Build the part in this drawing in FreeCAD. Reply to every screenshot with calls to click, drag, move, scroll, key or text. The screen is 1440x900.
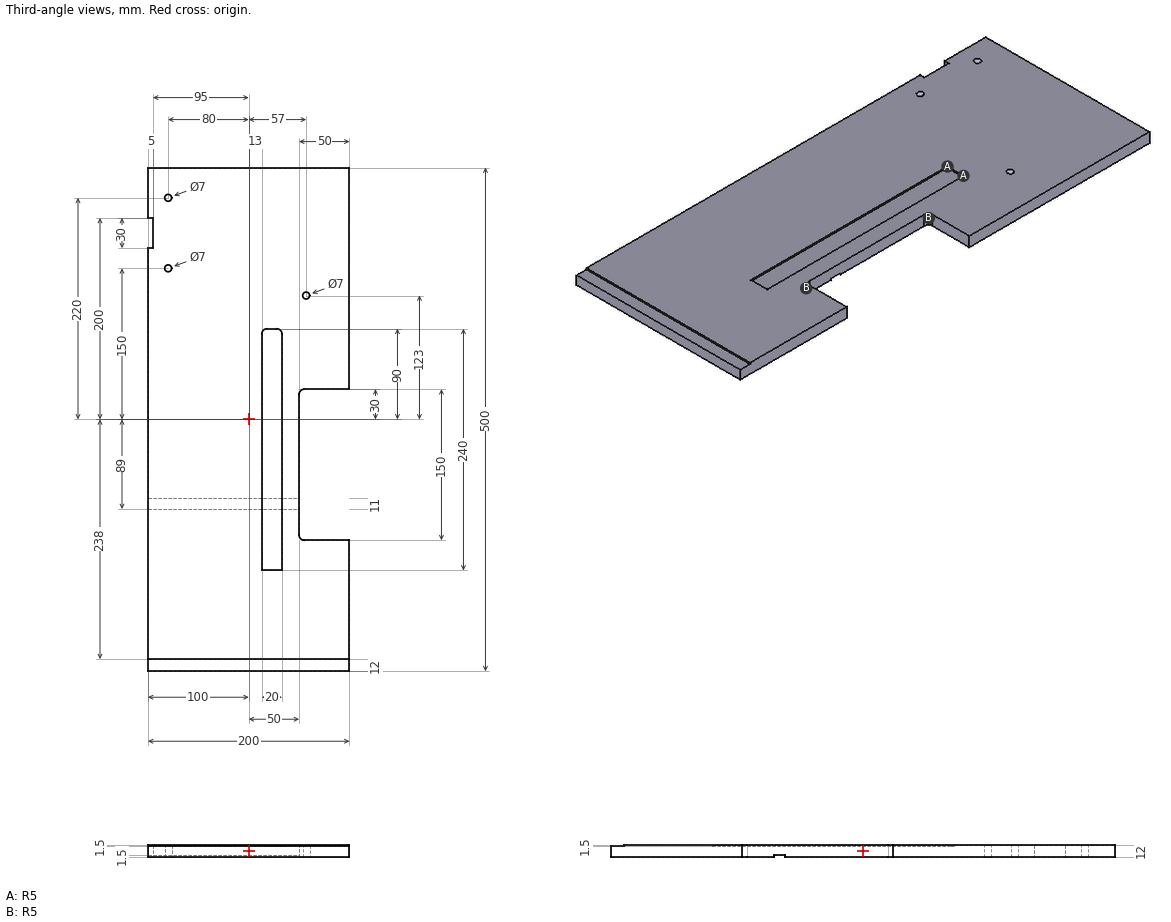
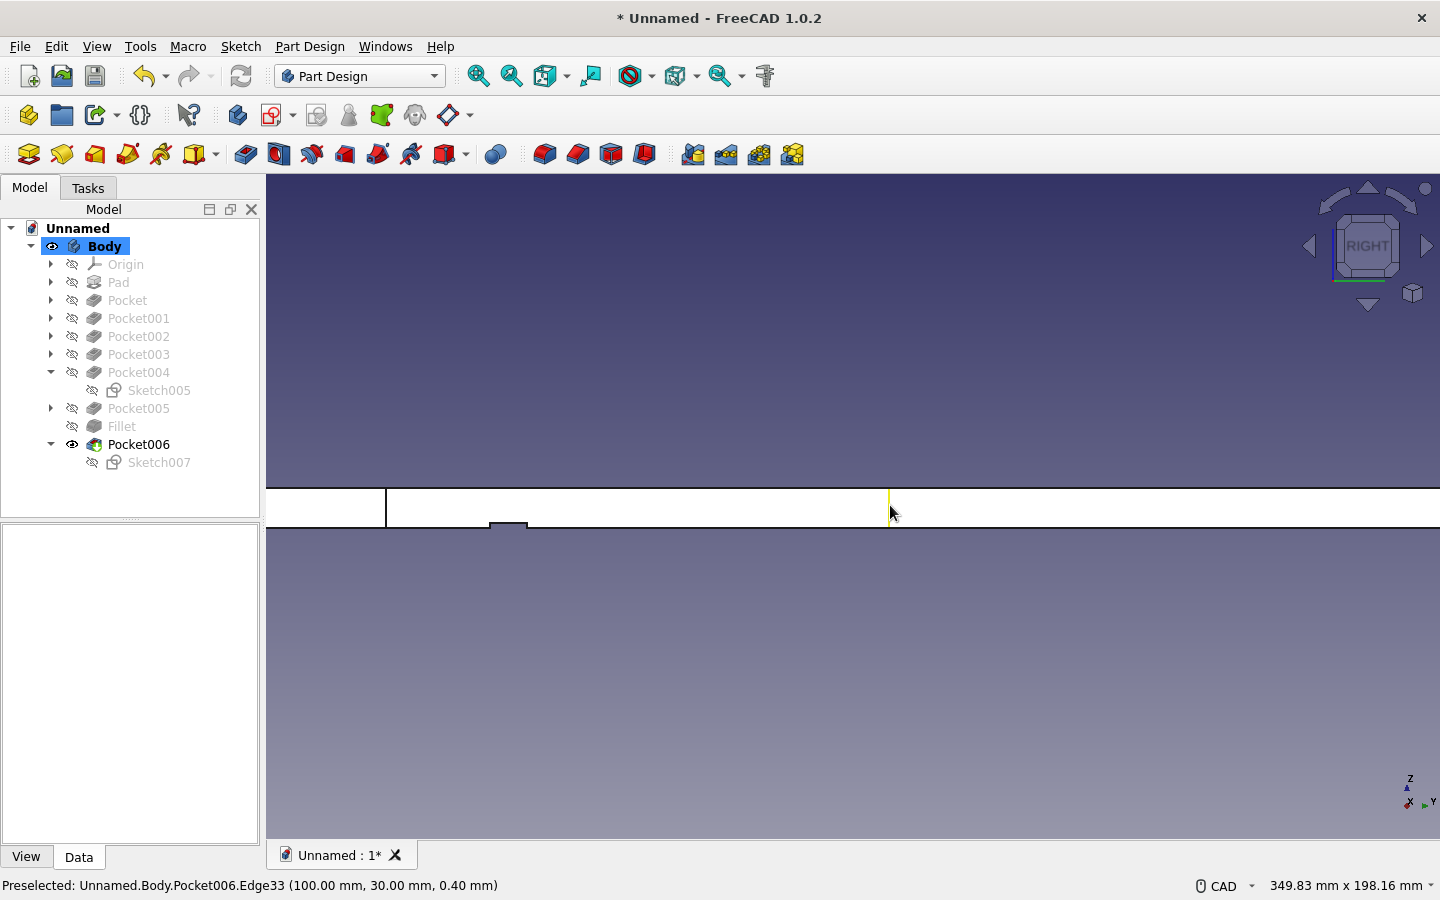
key(v)
key(f)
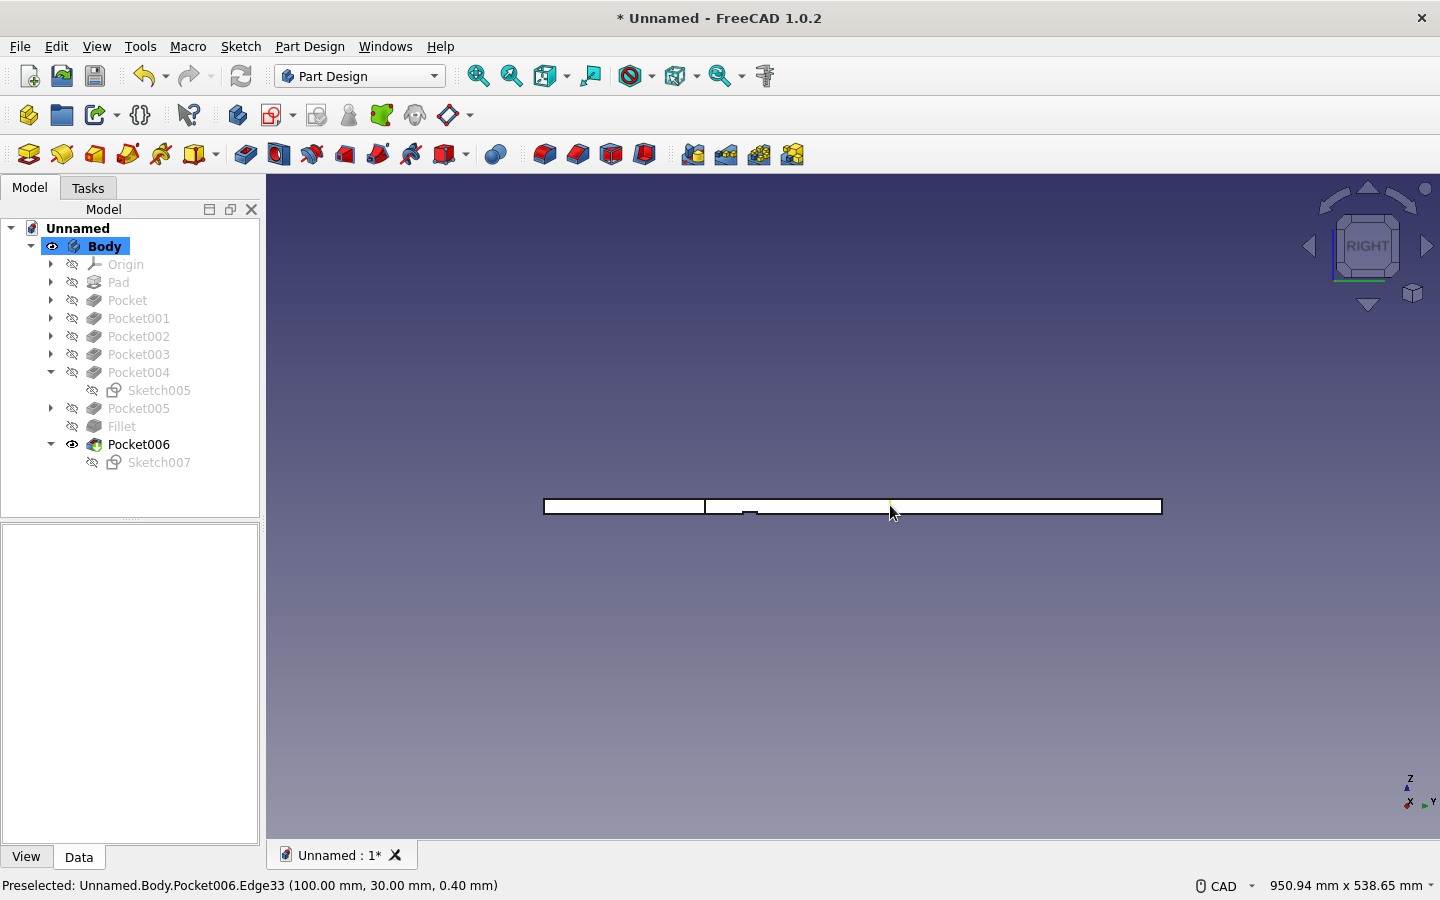
key(5)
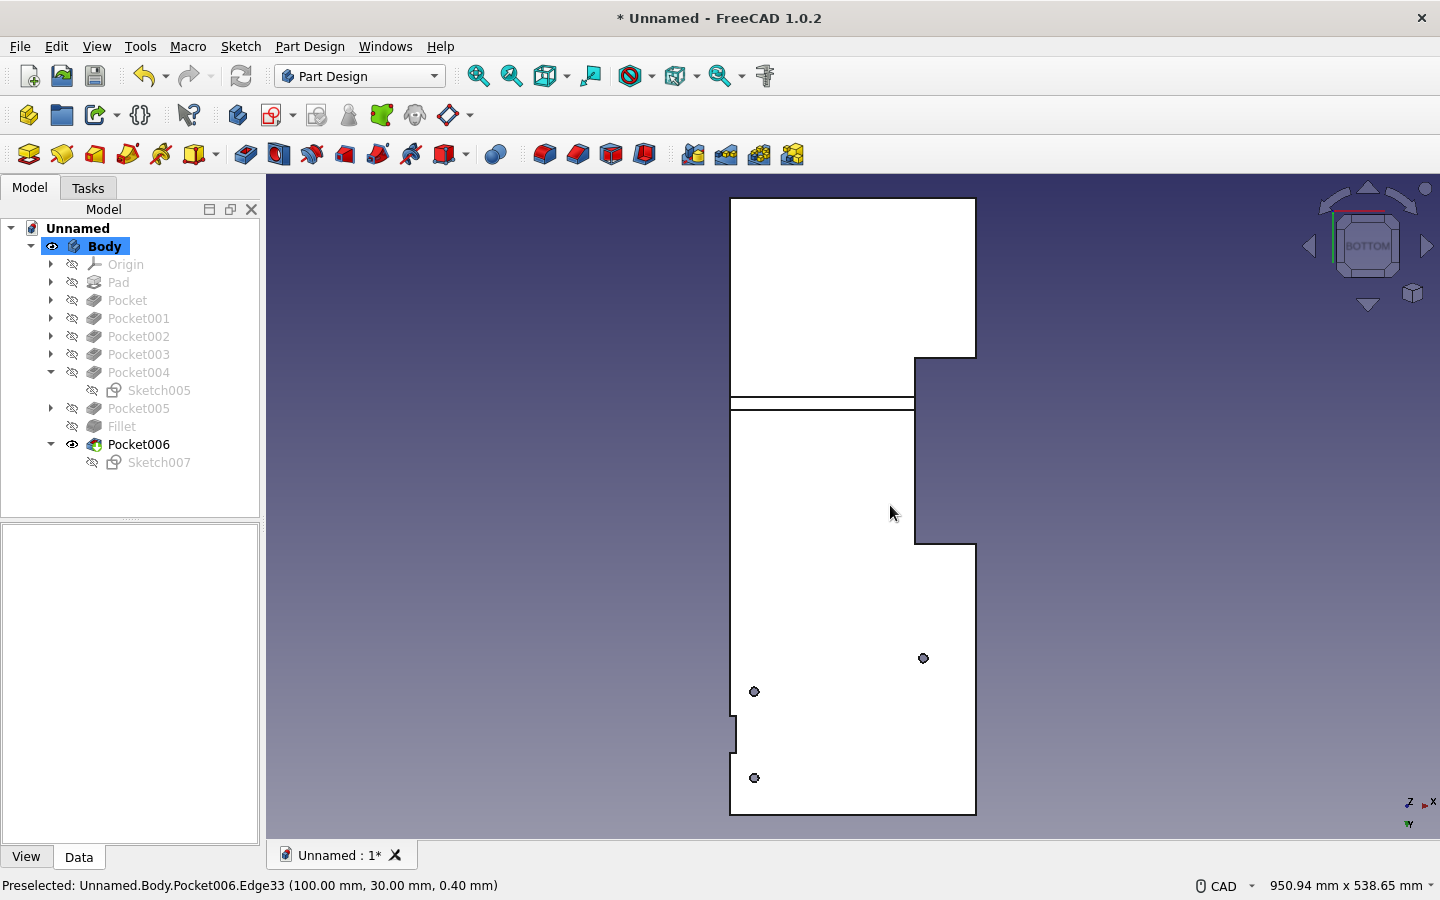
scroll(915, 543, up, 5)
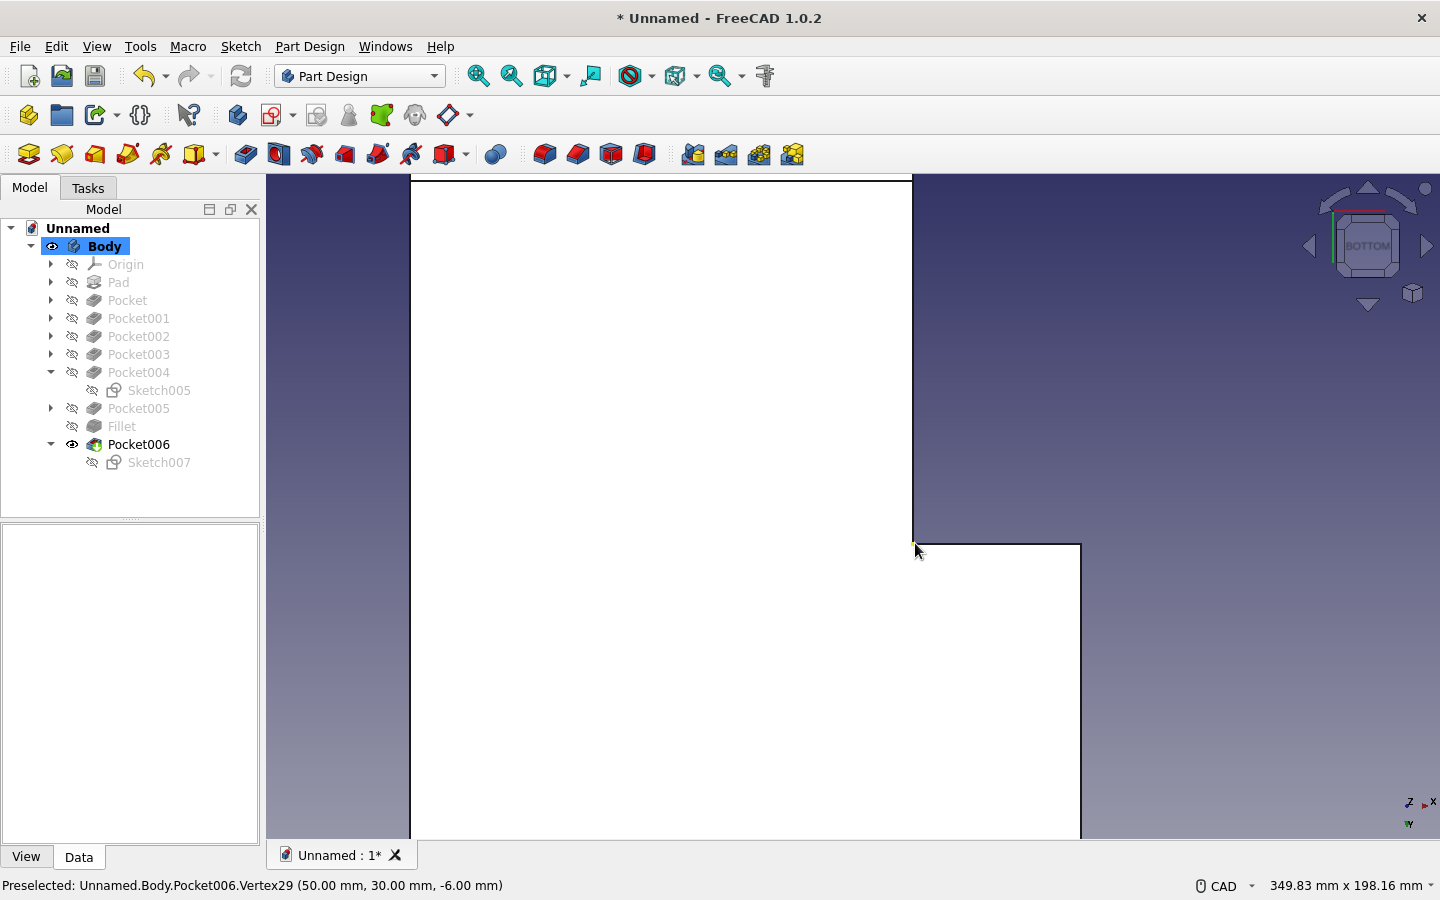
click(479, 76)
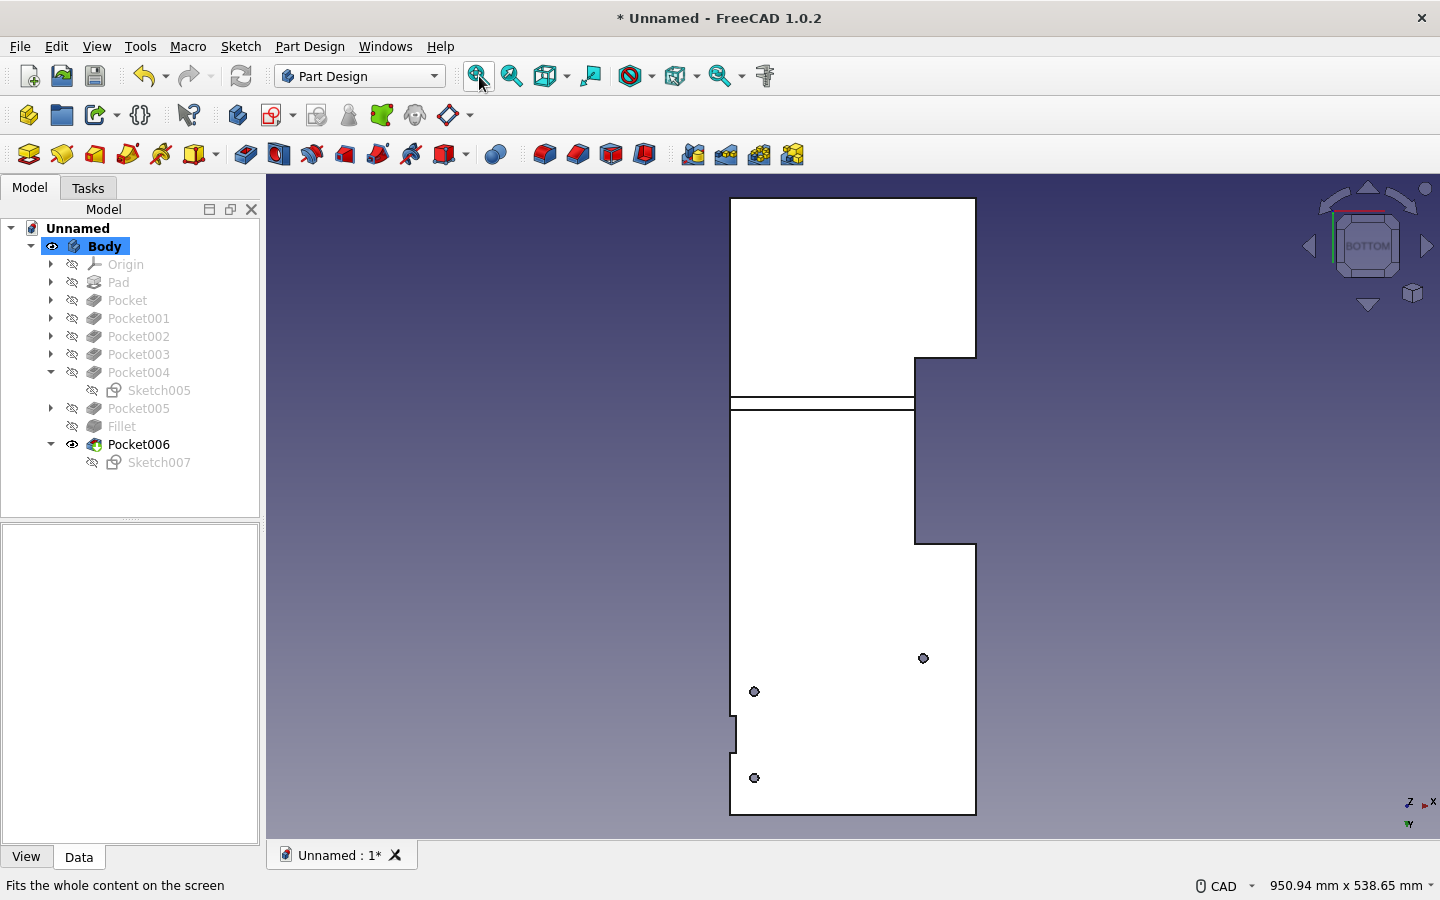
key(4)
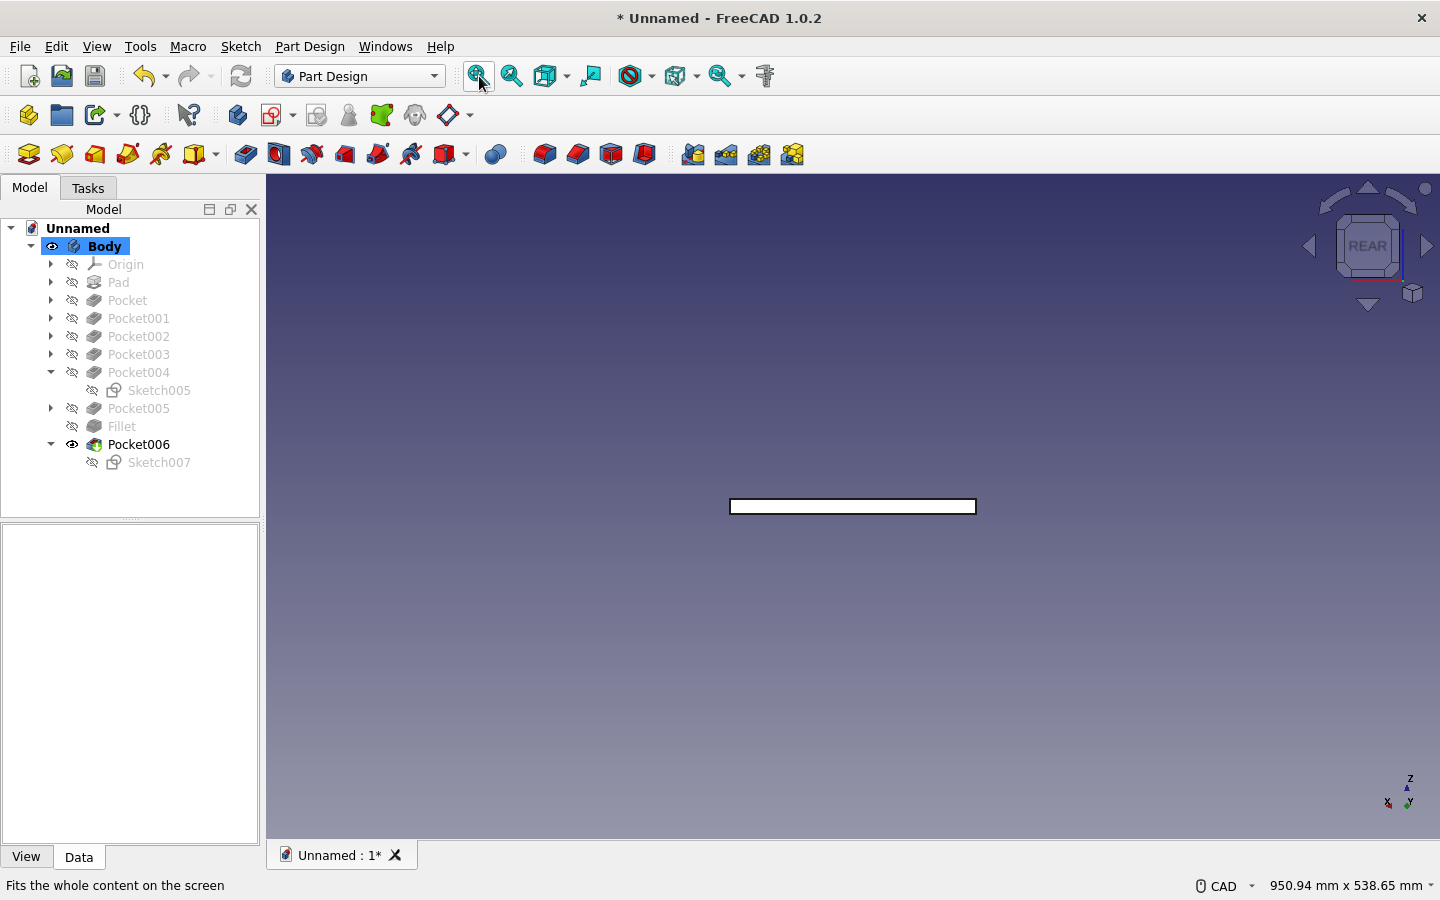
key(v)
key(f)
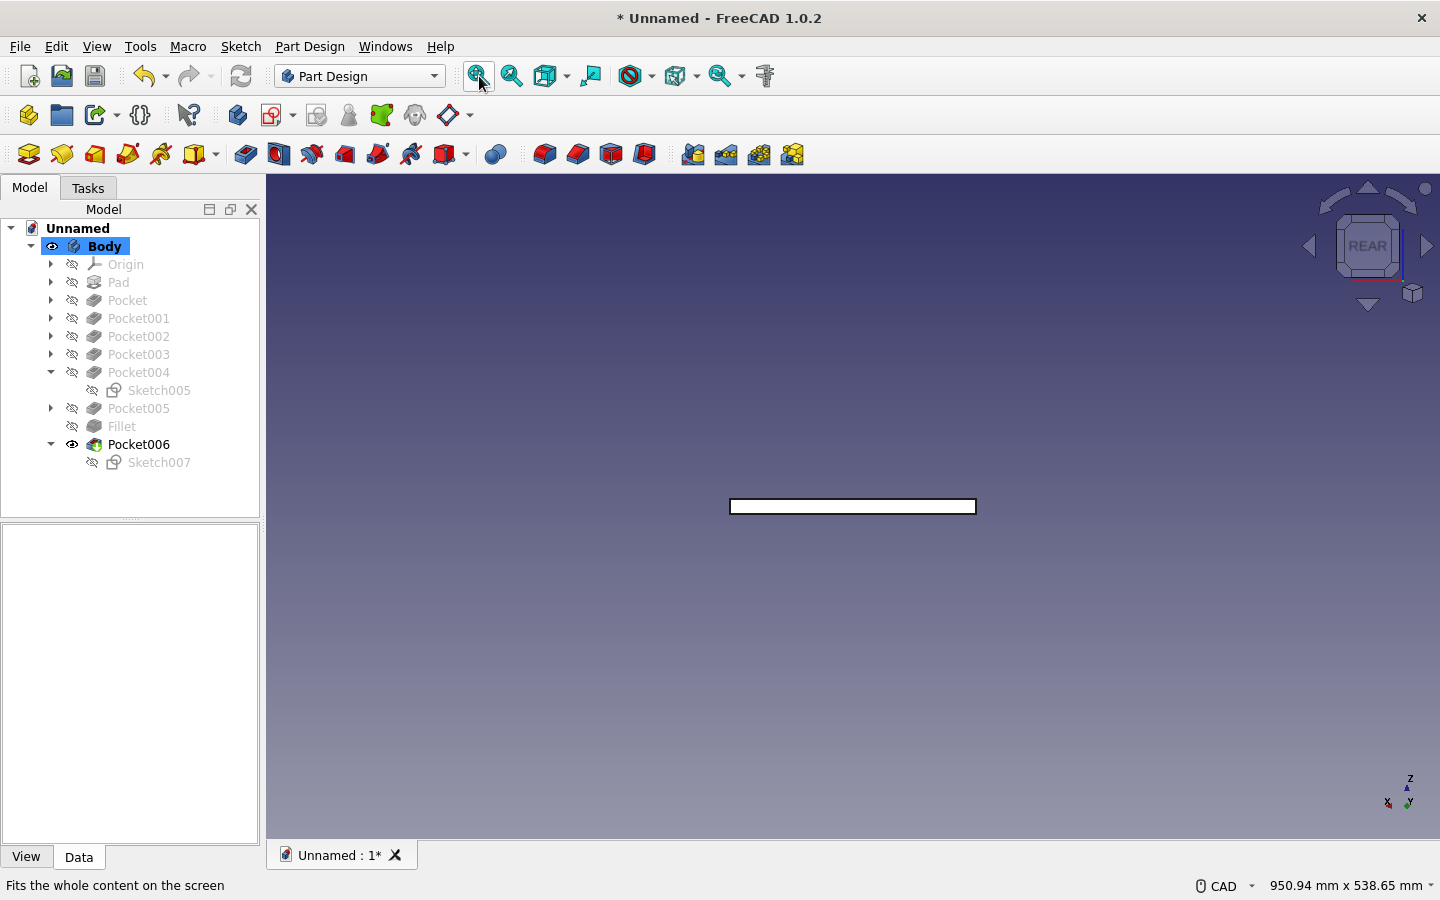
scroll(791, 506, up, 5)